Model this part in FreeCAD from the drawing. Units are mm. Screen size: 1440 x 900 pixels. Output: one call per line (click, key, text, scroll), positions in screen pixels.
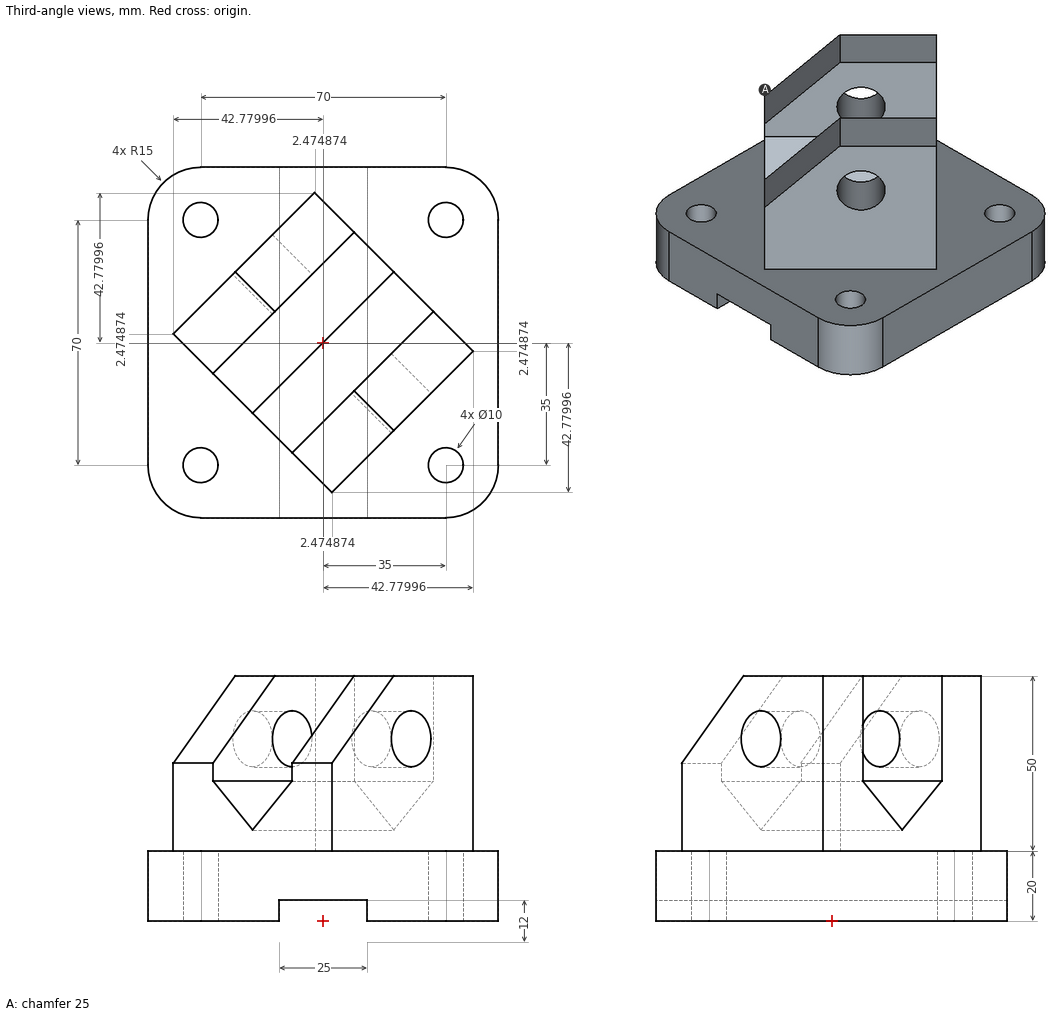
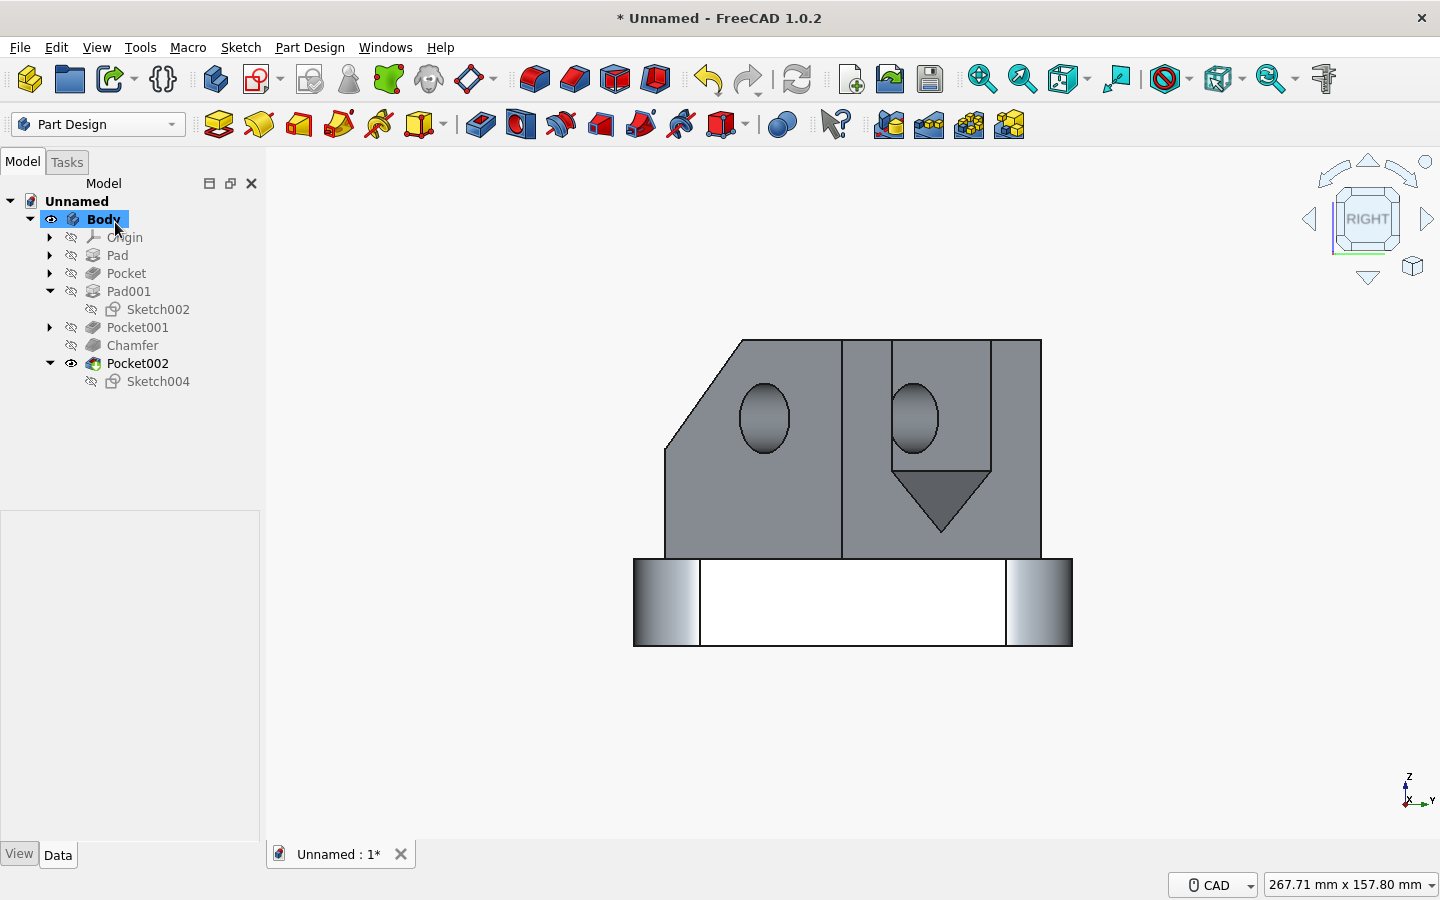
key(0)